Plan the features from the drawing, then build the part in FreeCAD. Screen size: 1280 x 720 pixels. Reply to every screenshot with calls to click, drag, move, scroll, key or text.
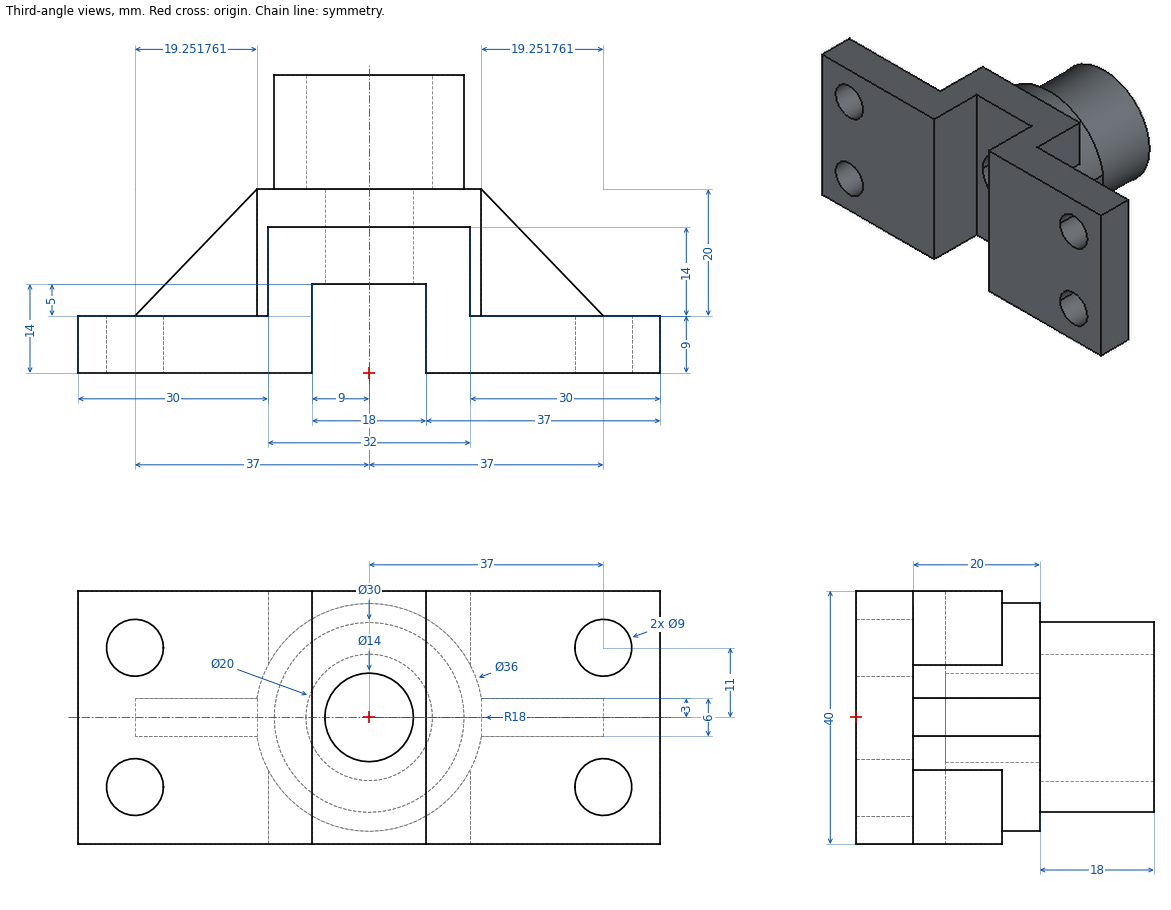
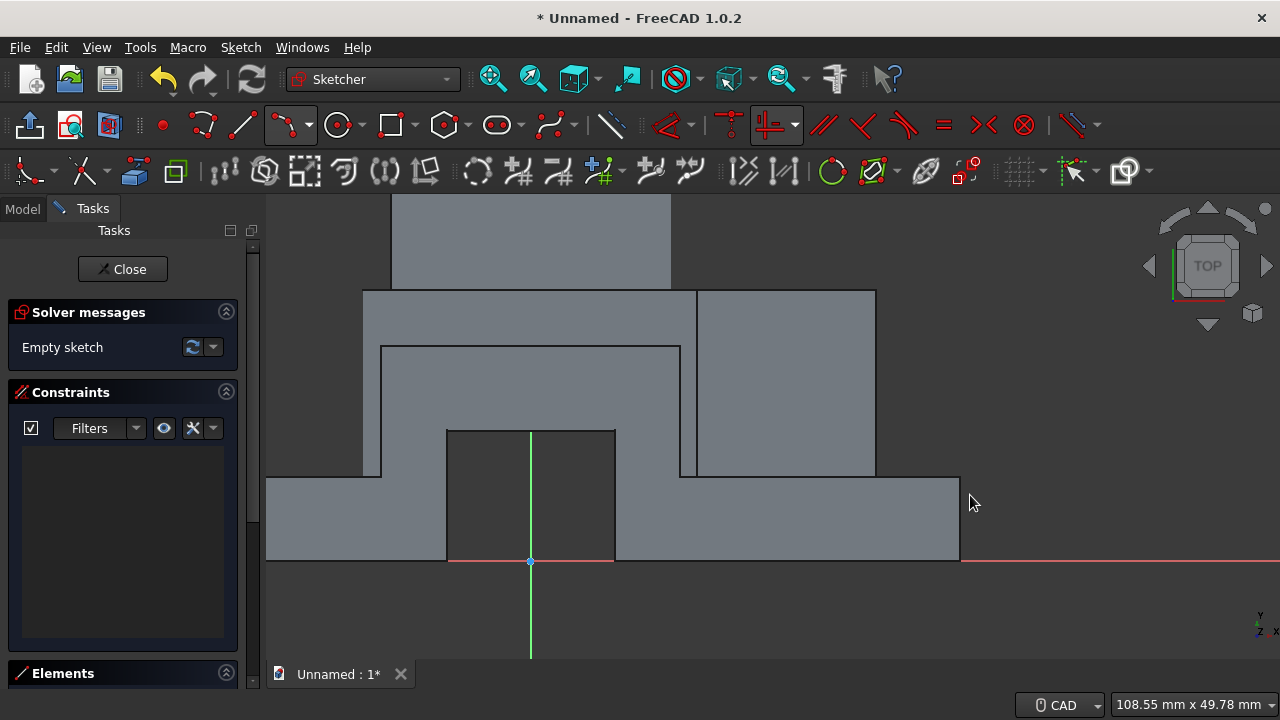
key(g)
key(m)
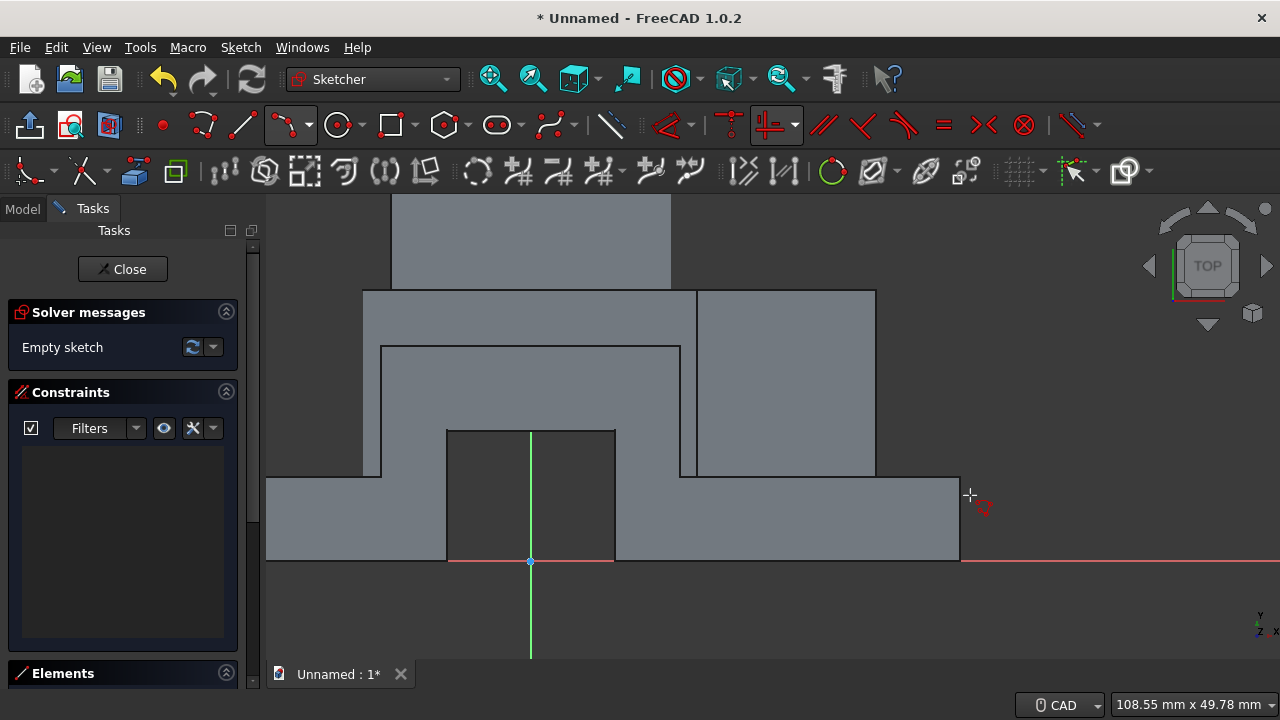
click(697, 290)
click(876, 477)
click(876, 290)
click(697, 291)
key(Escape)
key(Escape)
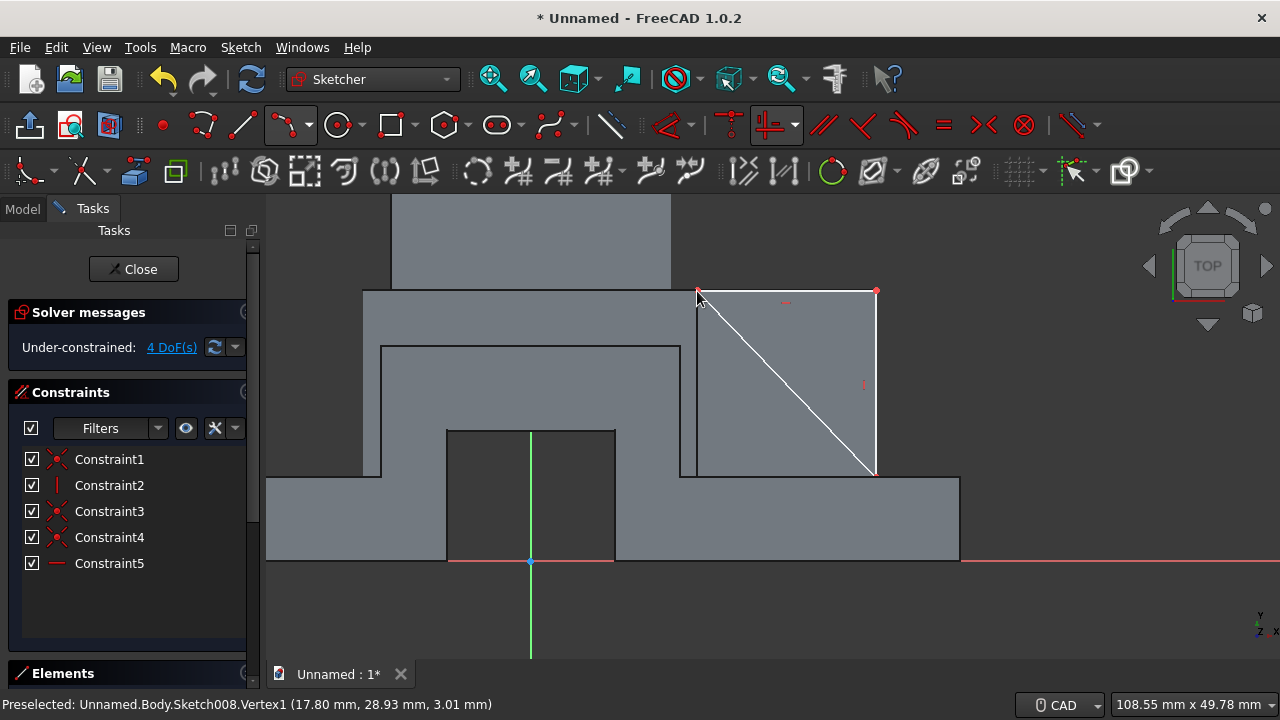
click(666, 126)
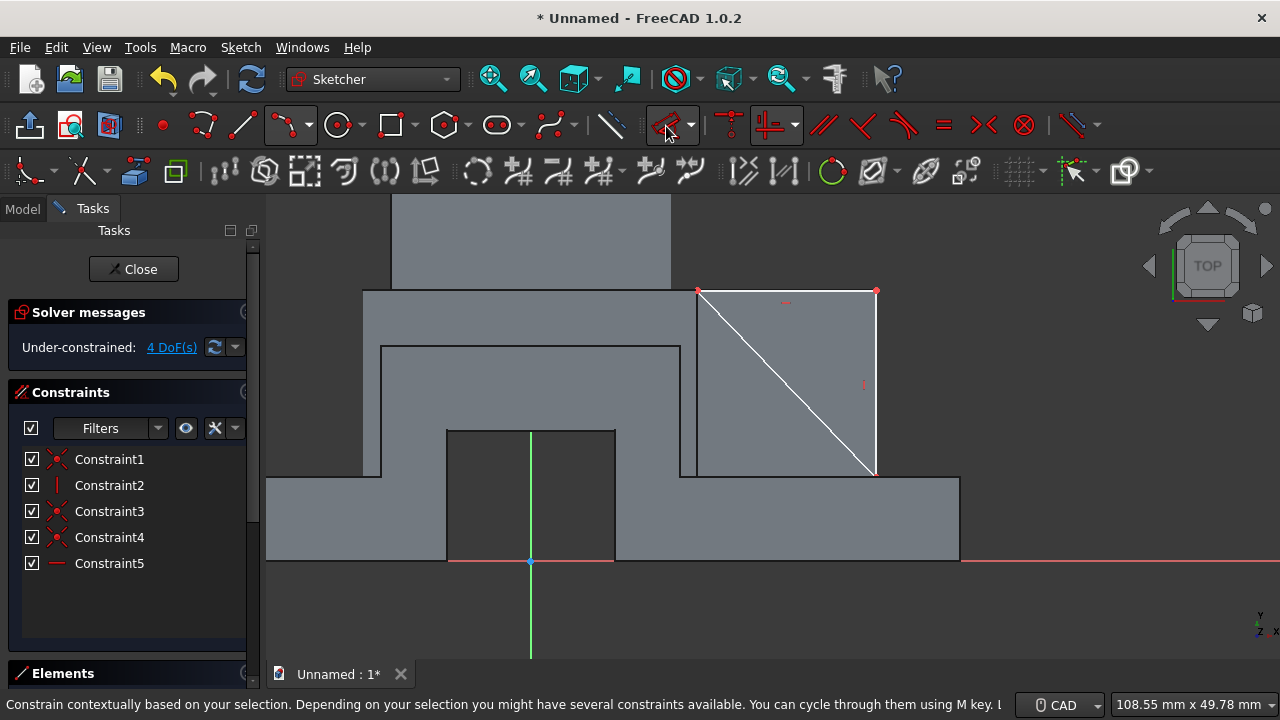
click(876, 422)
click(910, 384)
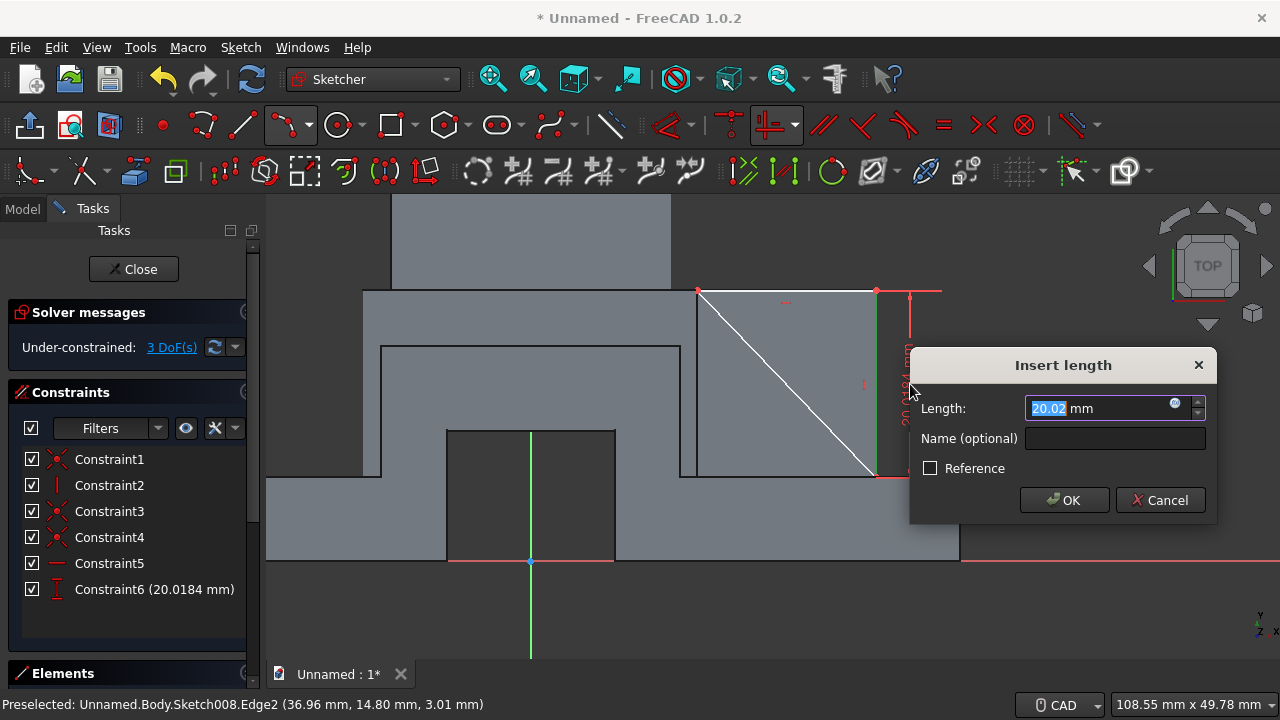
text(20)
key(Return)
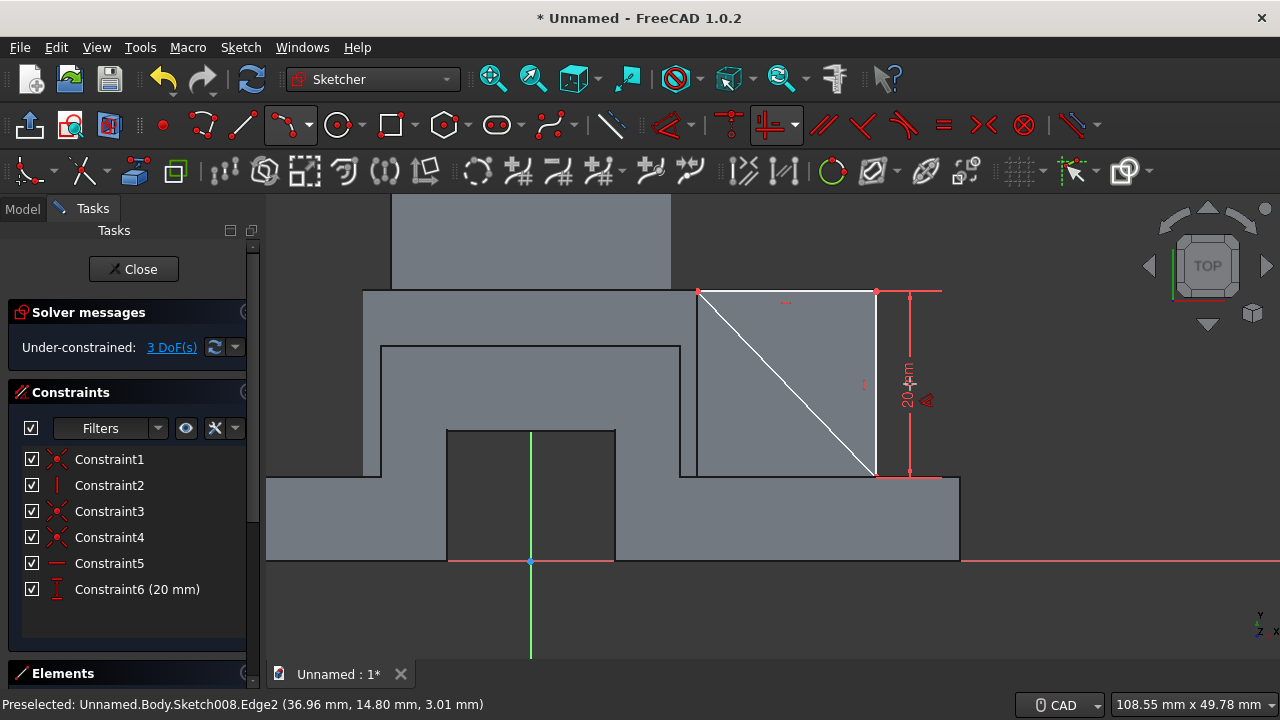
click(876, 478)
click(497, 520)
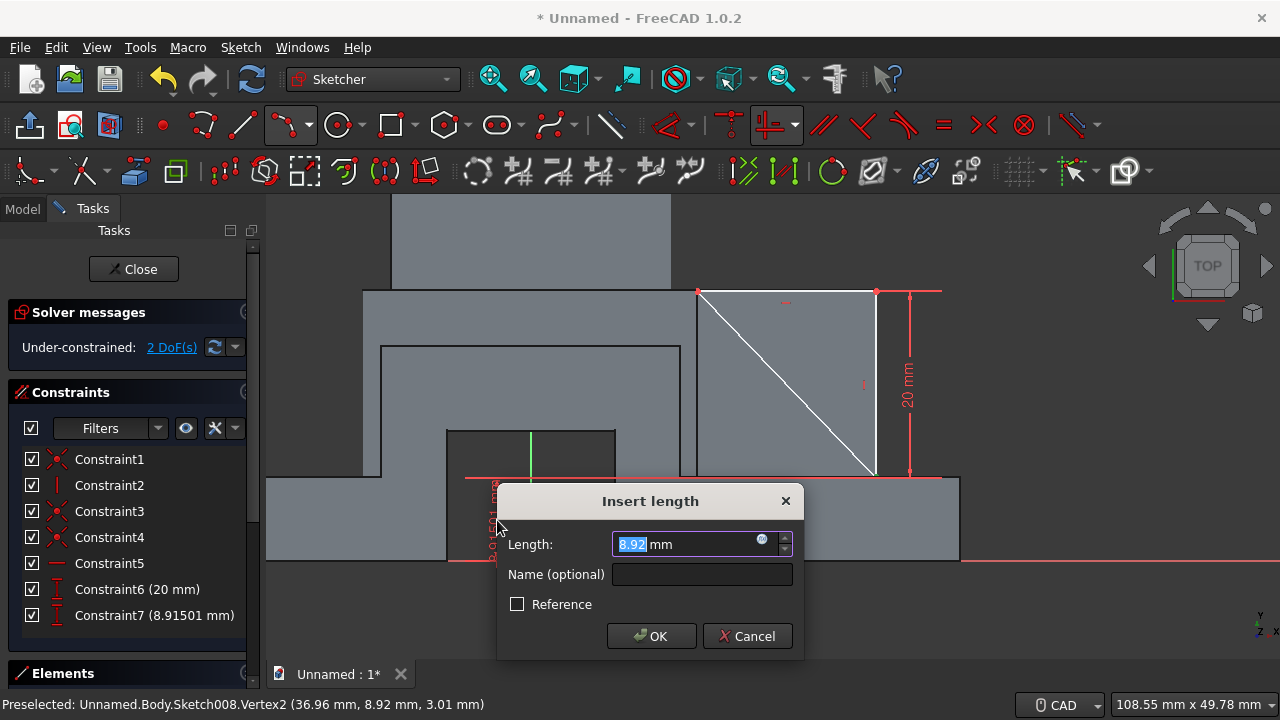
text(9)
key(Return)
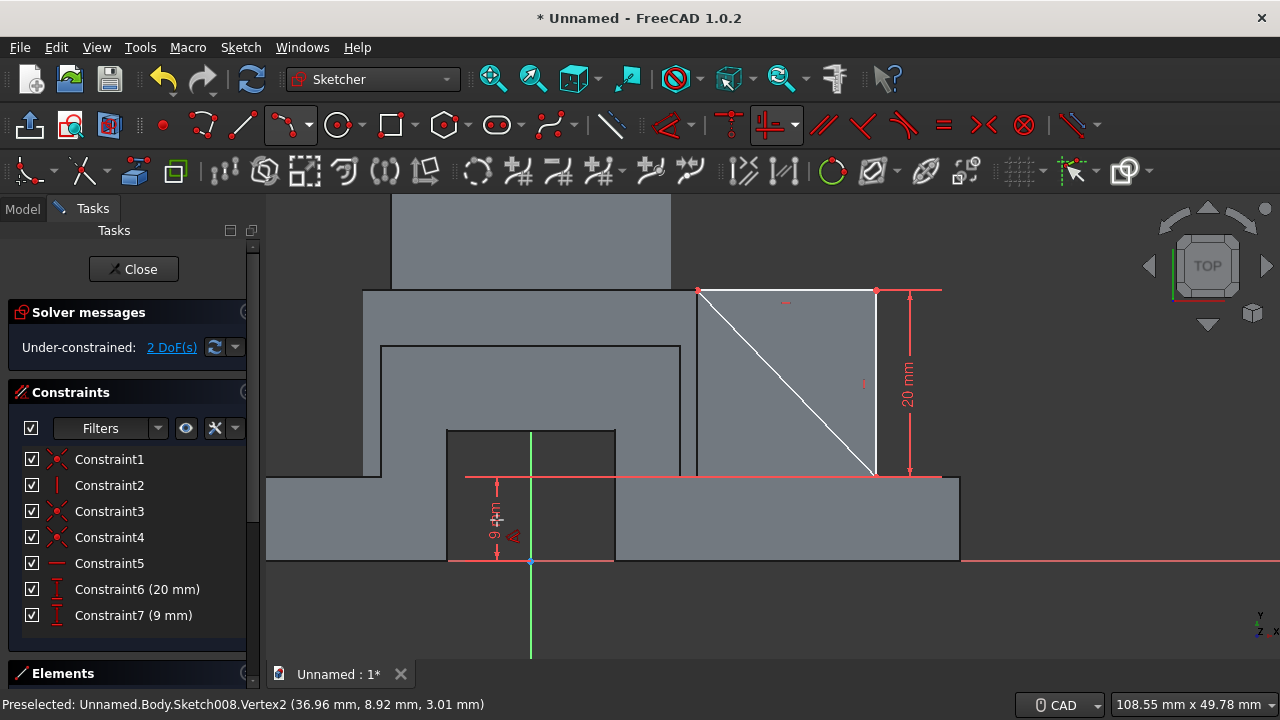
click(876, 477)
click(703, 595)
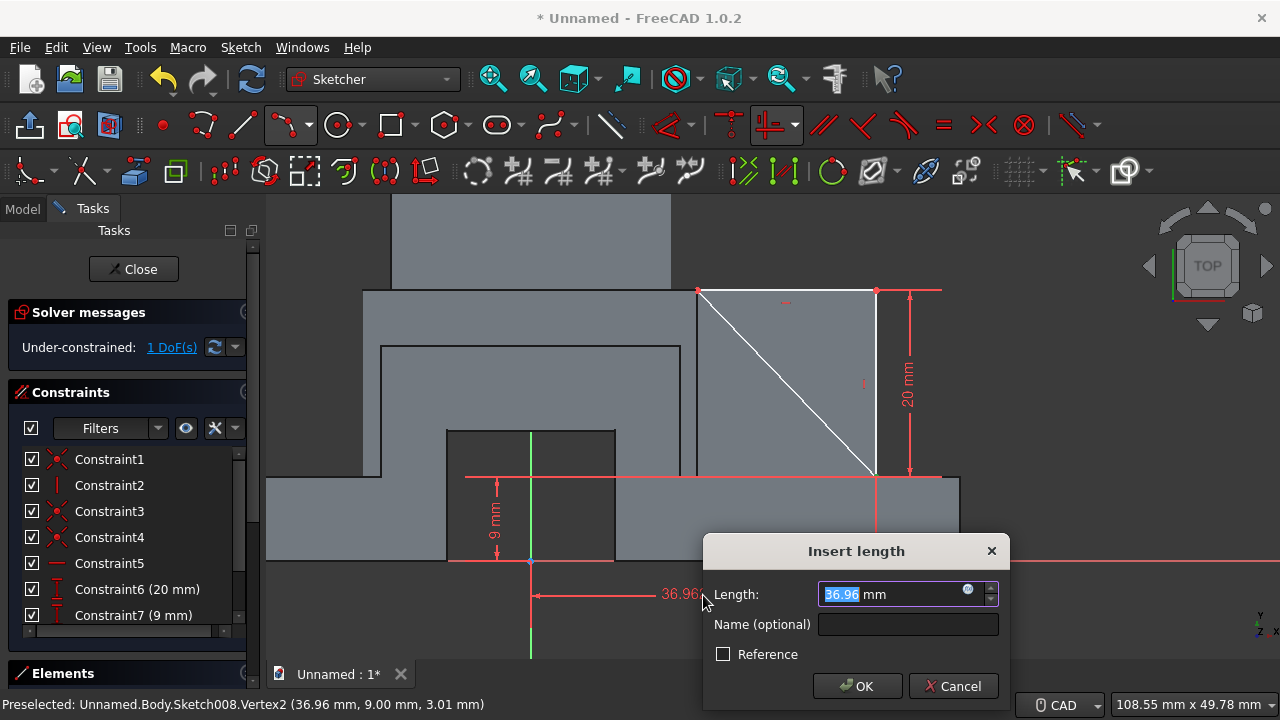
text(37)
key(Return)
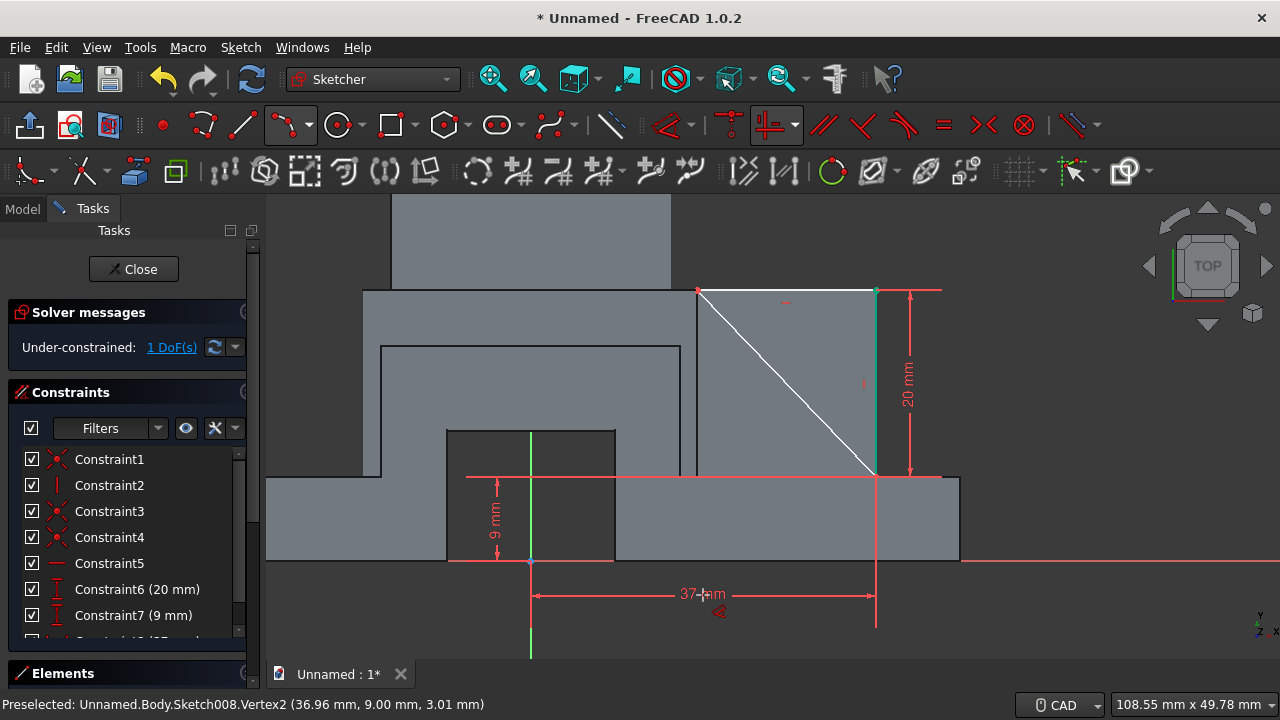
click(823, 290)
click(787, 256)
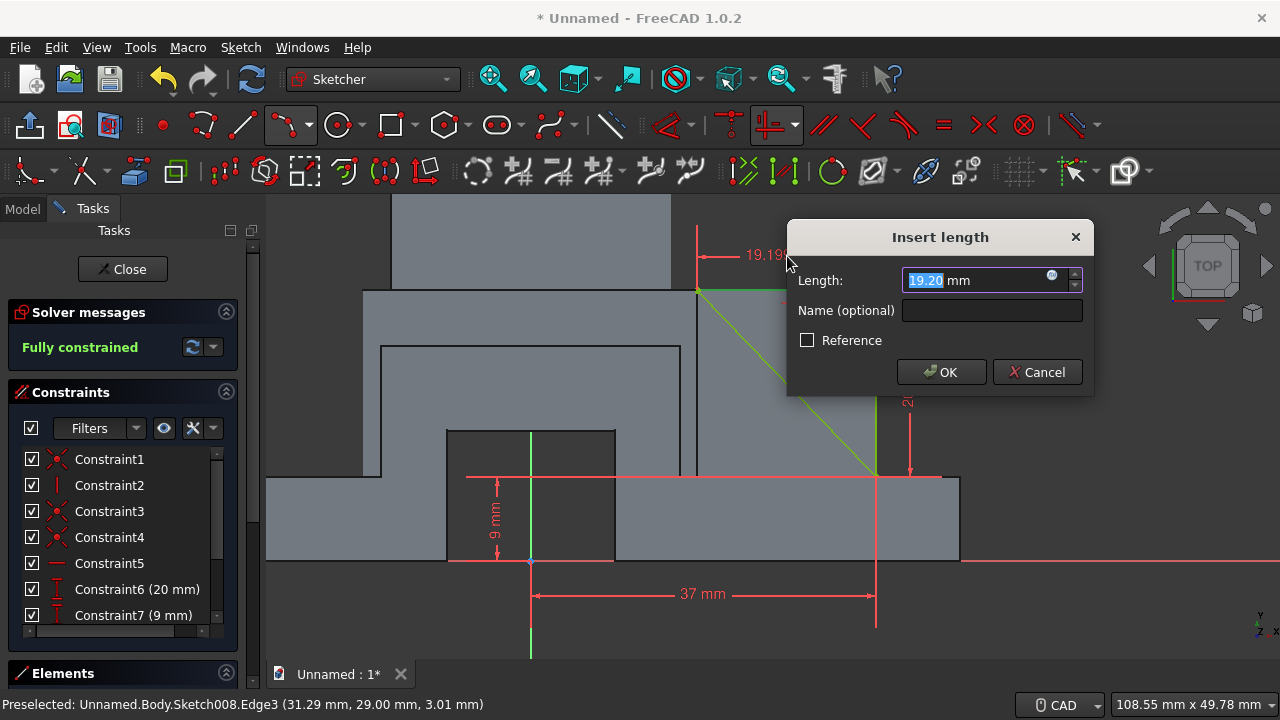
text(19.251761)
key(Return)
key(Escape)